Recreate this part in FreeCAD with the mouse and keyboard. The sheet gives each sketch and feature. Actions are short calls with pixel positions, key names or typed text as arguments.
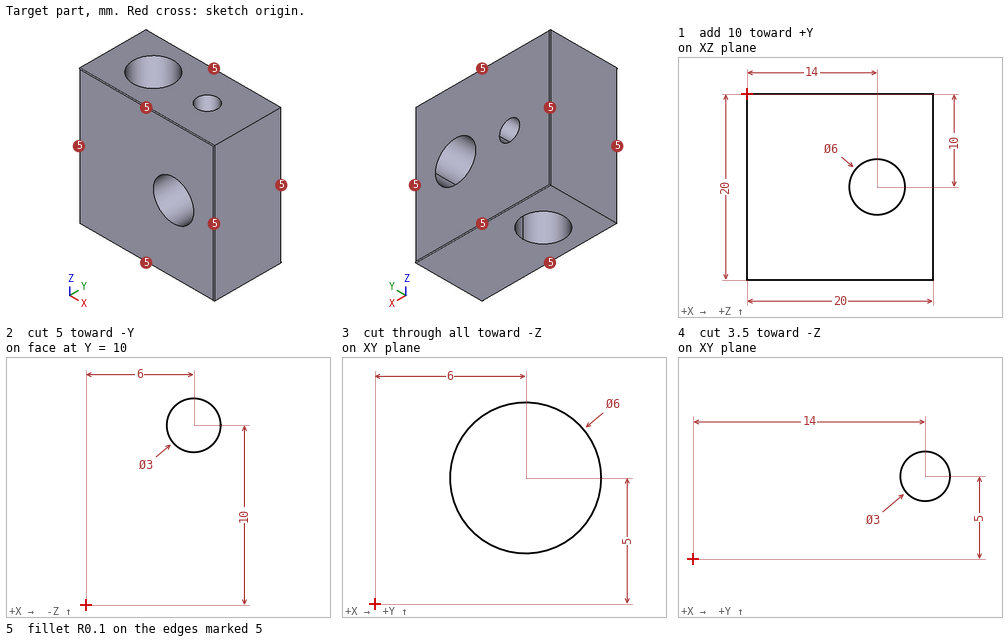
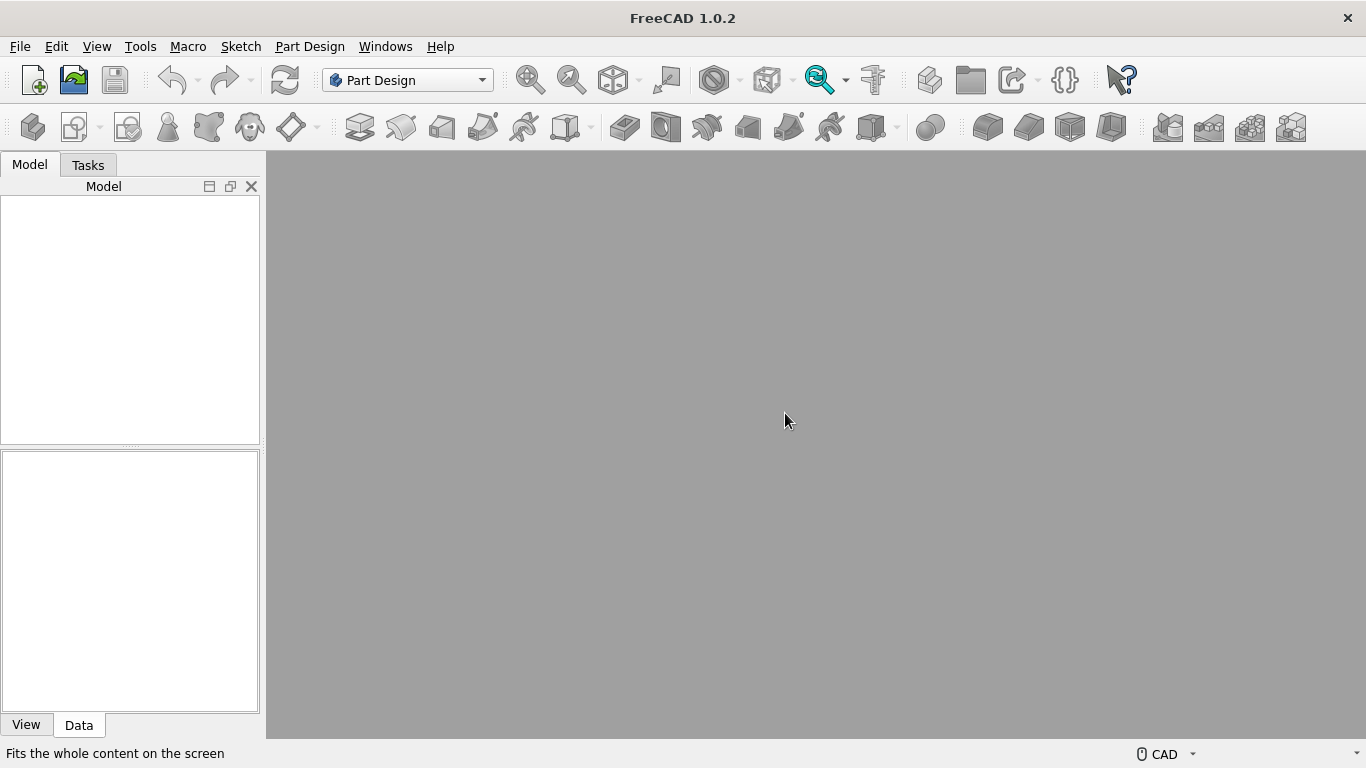
key(ctrl+n)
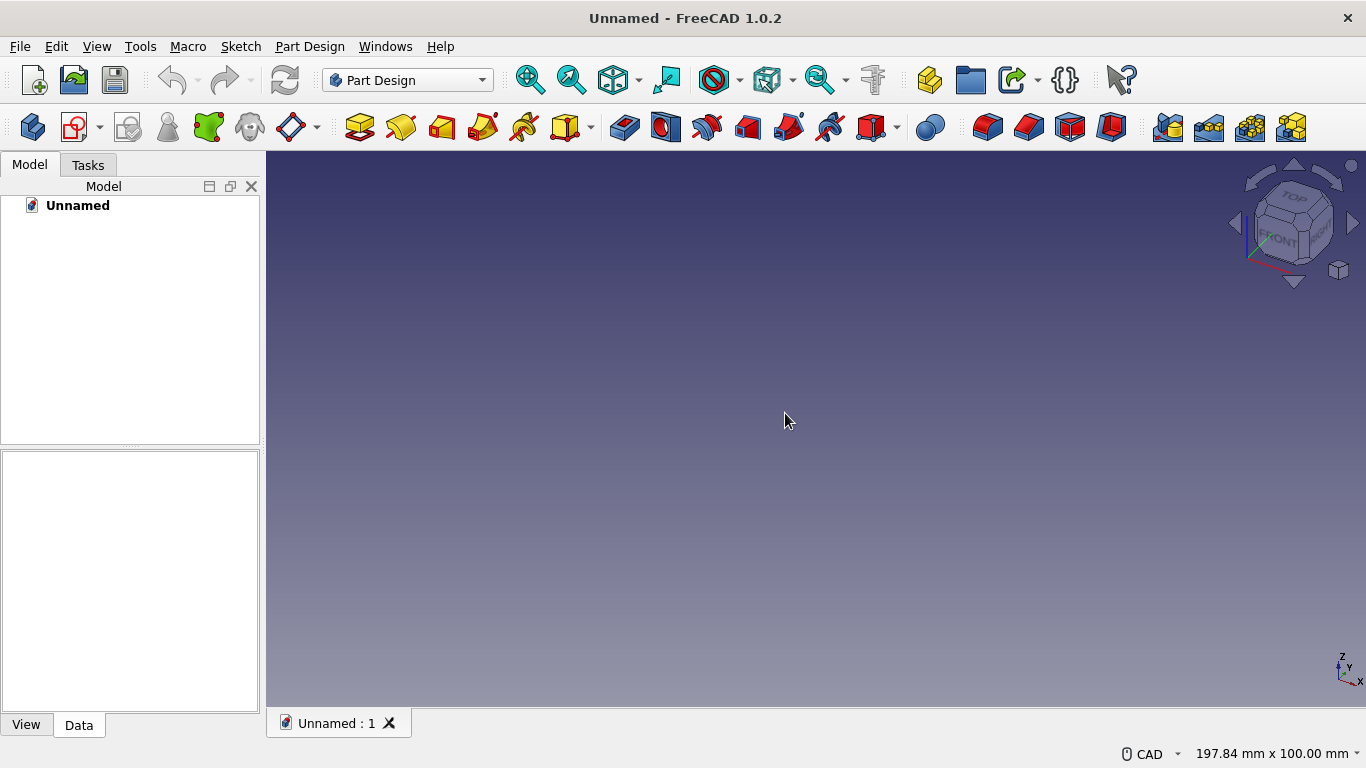
click(74, 128)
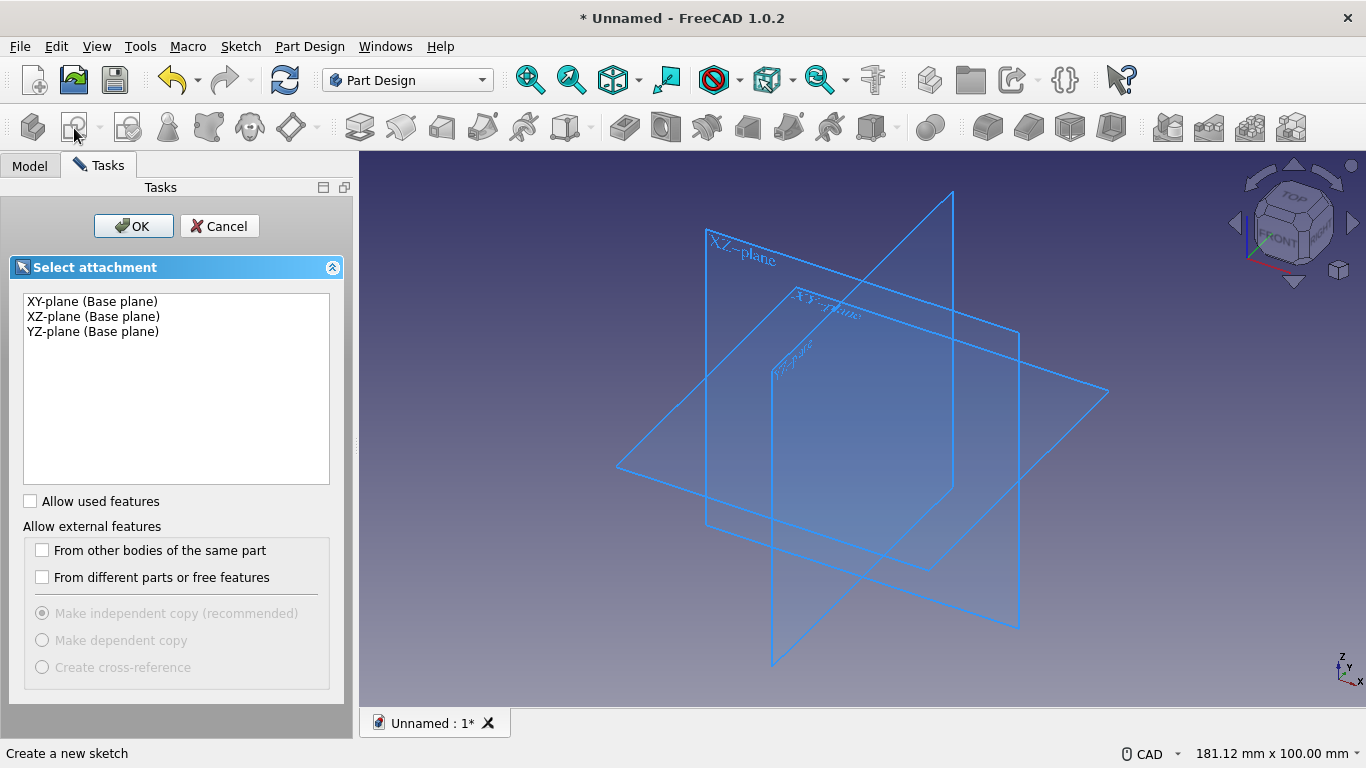
click(84, 316)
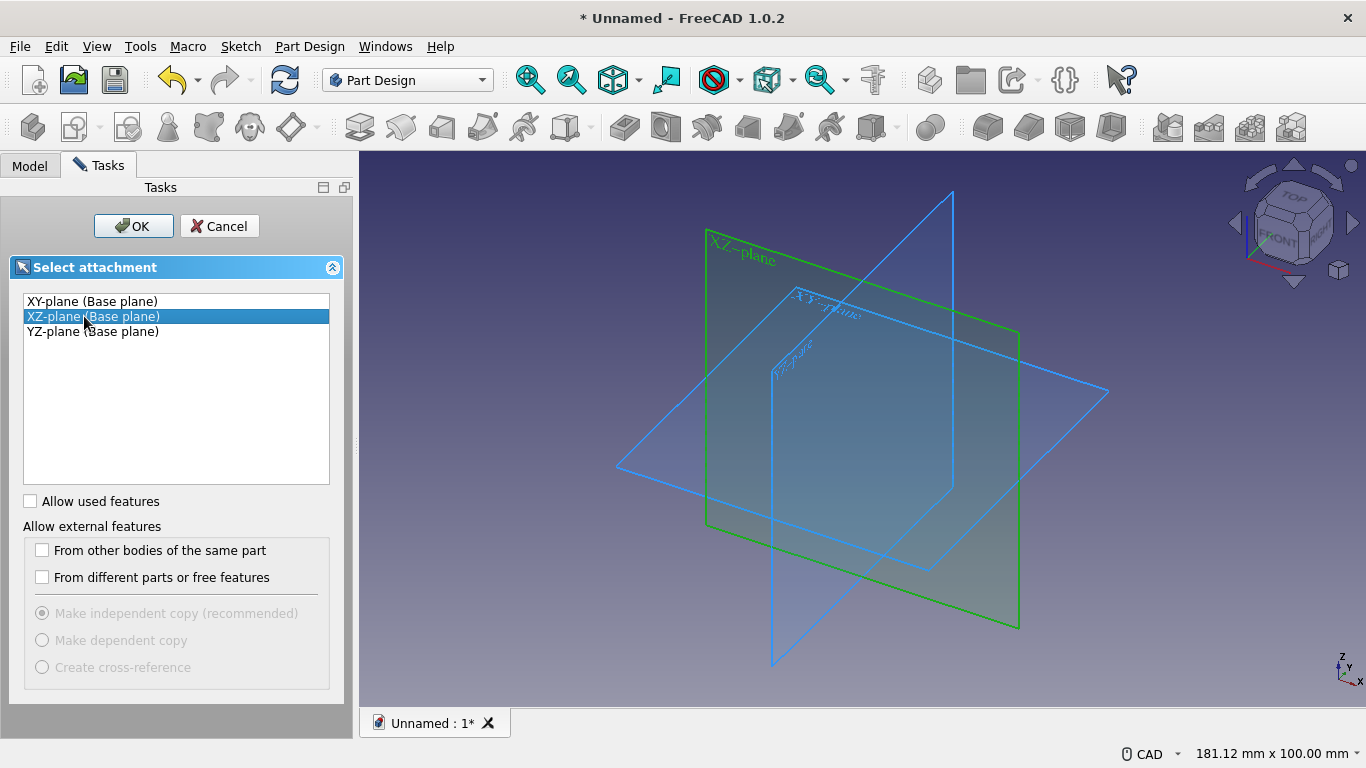
click(134, 226)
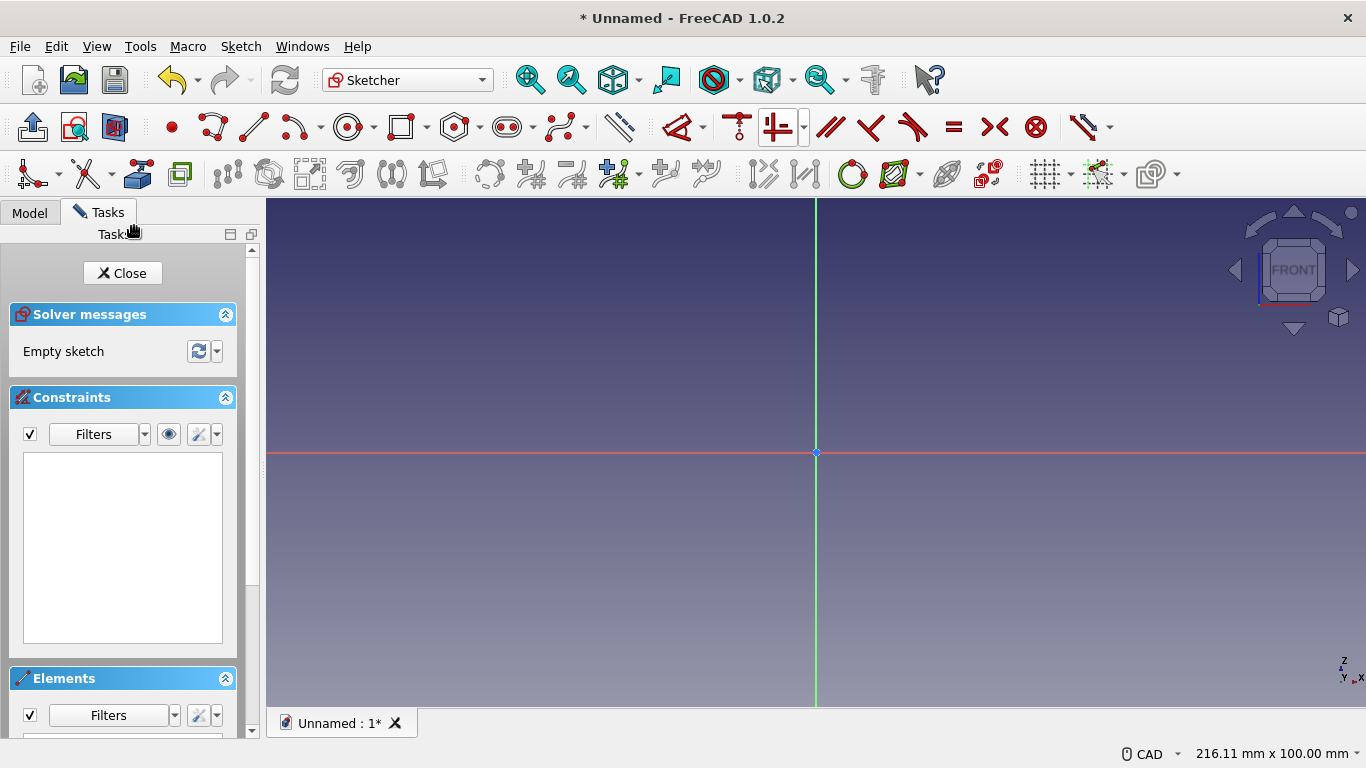
scroll(918, 525, up, 6)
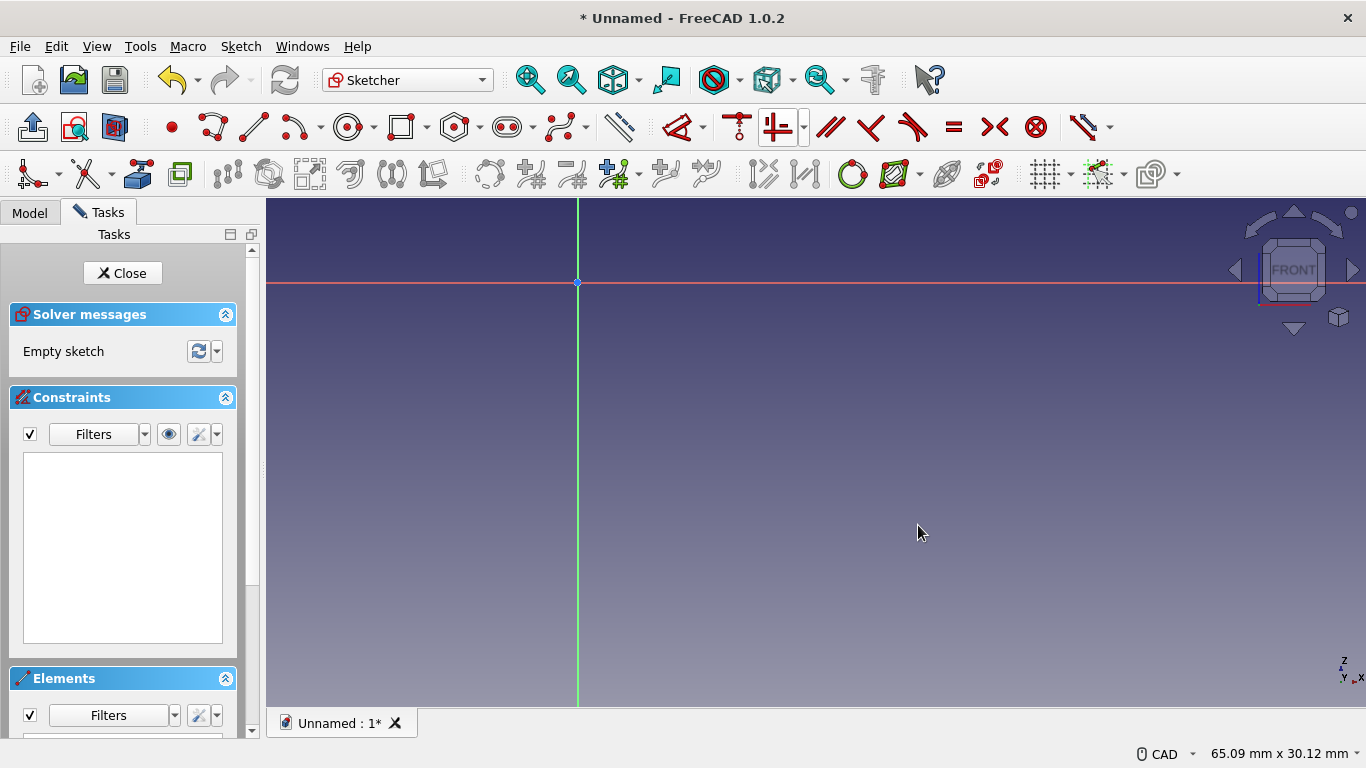
click(400, 128)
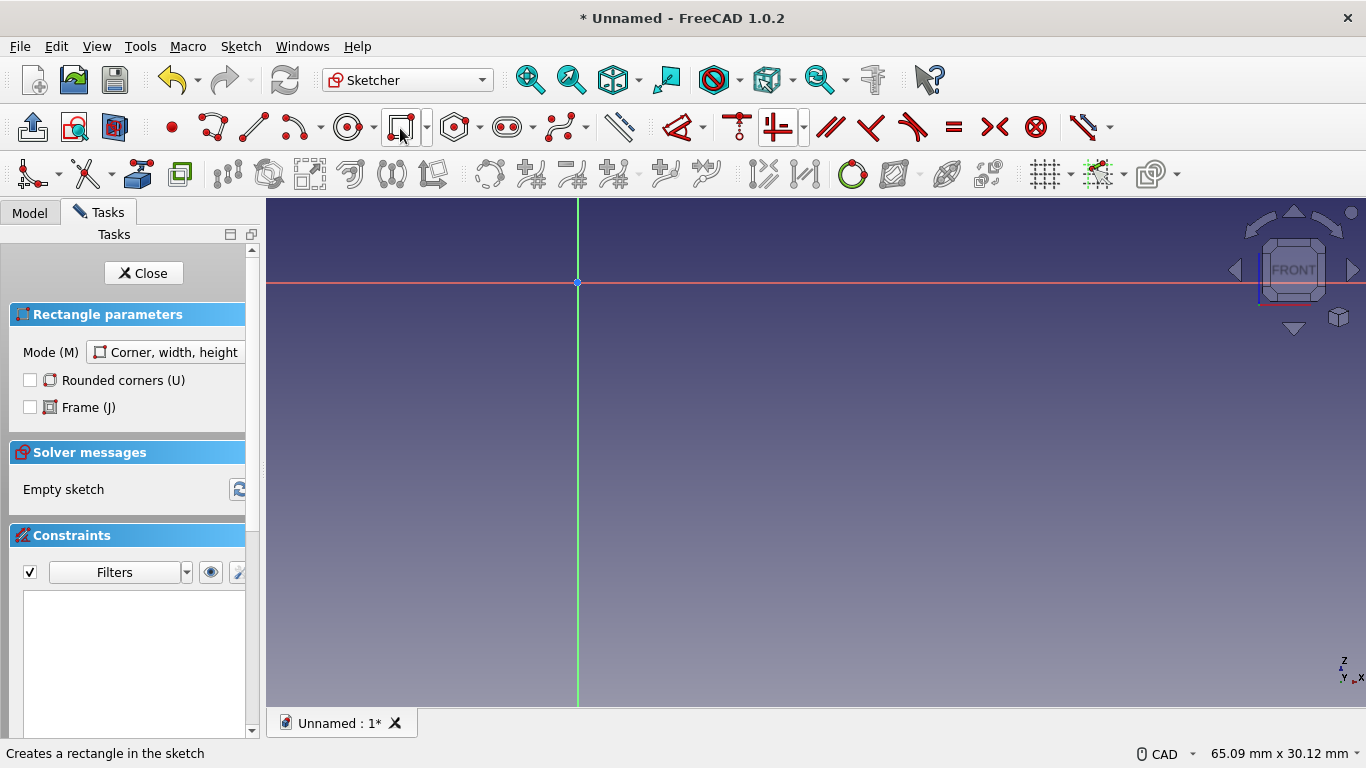
click(578, 283)
click(916, 621)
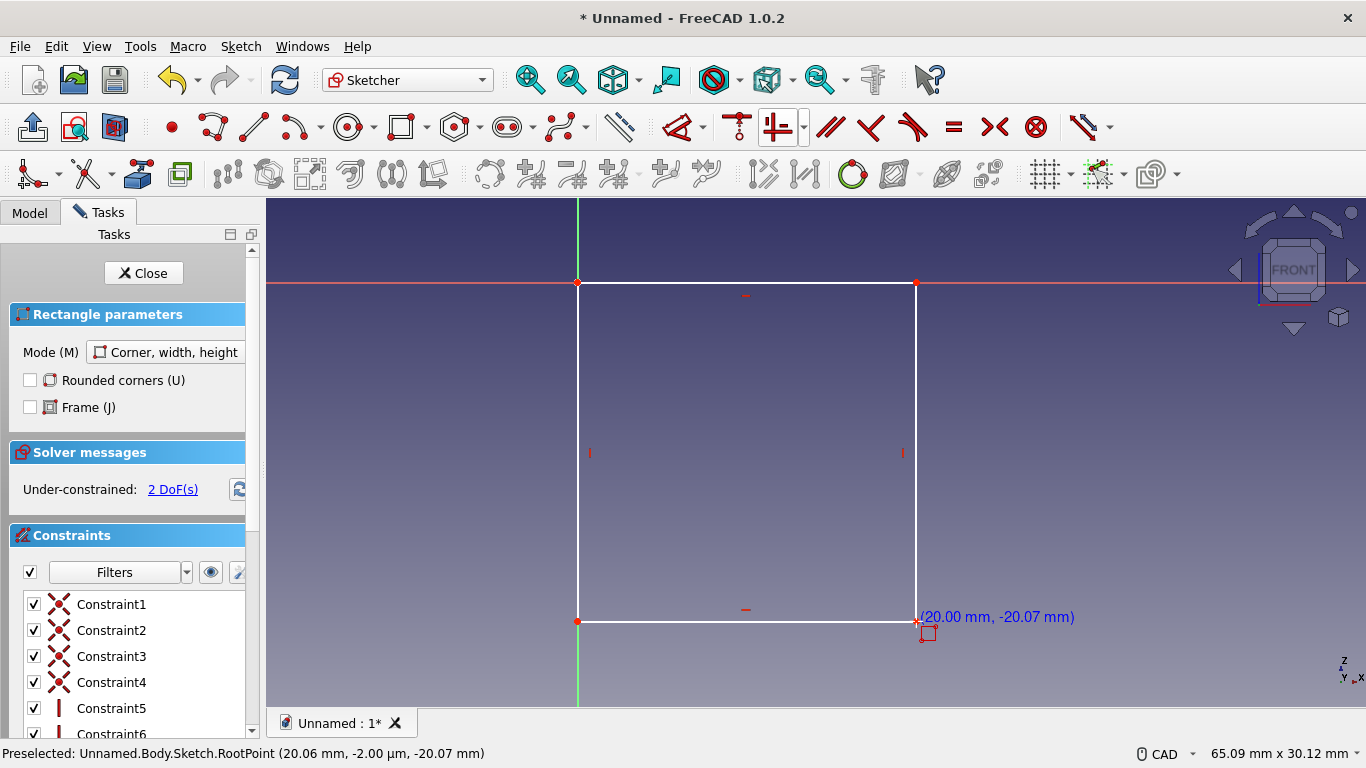
key(g)
key(c)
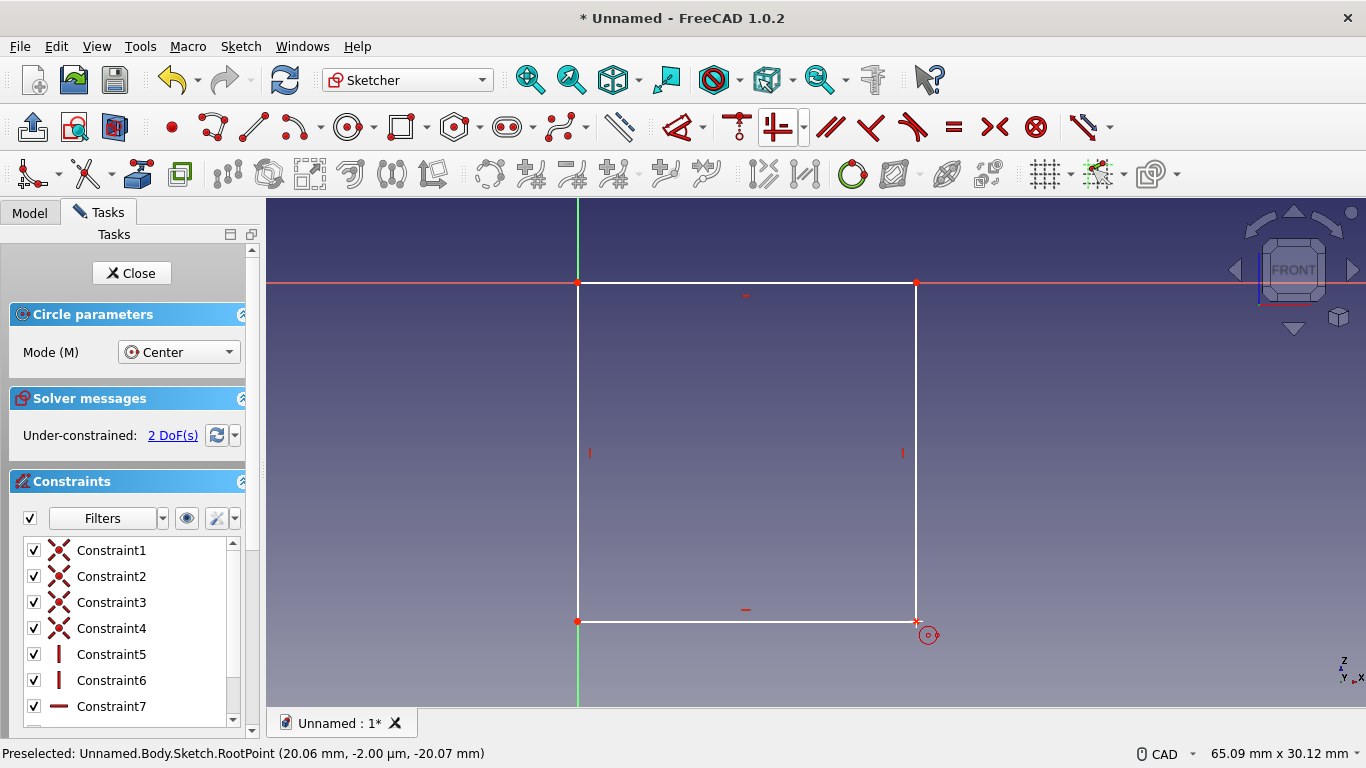
click(815, 452)
click(850, 416)
key(Escape)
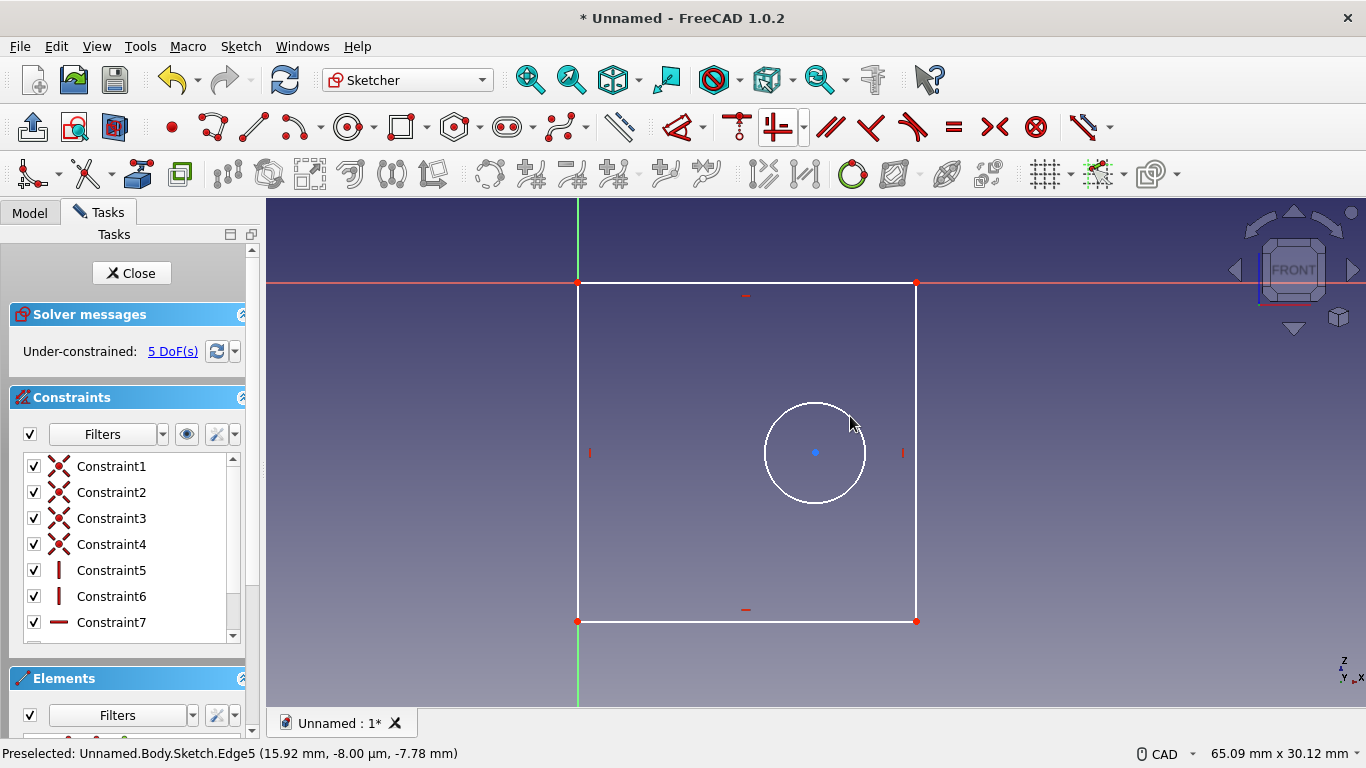
key(d)